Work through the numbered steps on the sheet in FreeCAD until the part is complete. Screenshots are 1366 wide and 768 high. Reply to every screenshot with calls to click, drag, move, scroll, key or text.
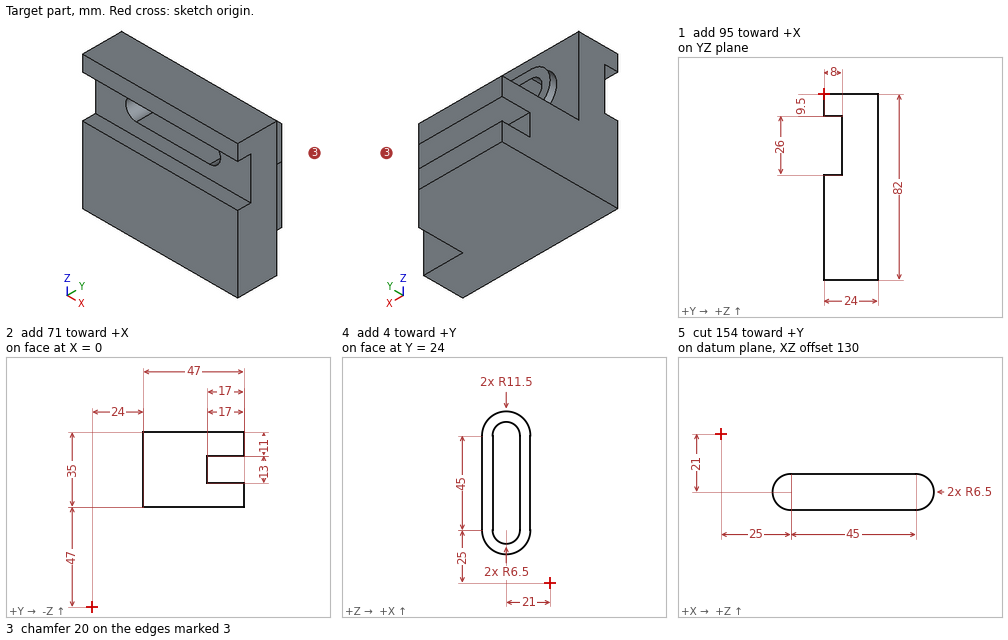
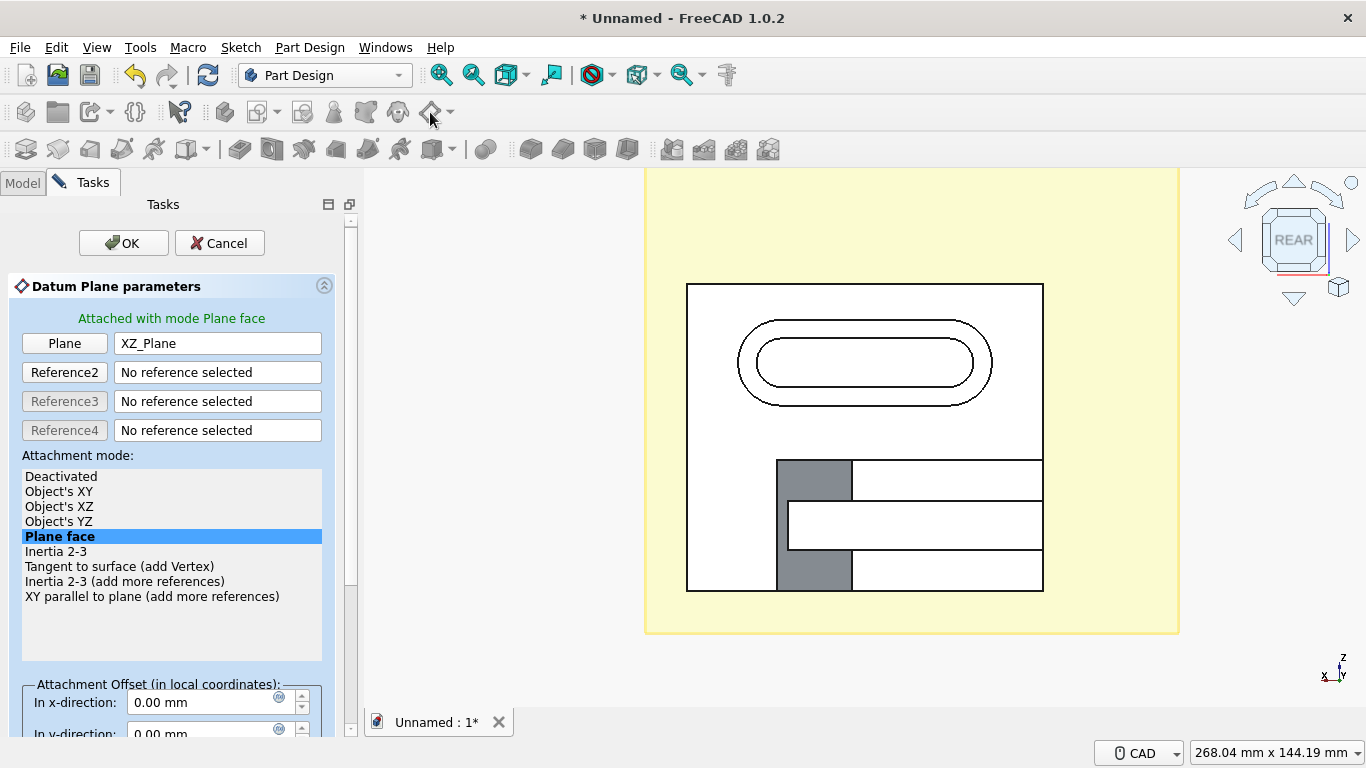
scroll(351, 475, down, 2)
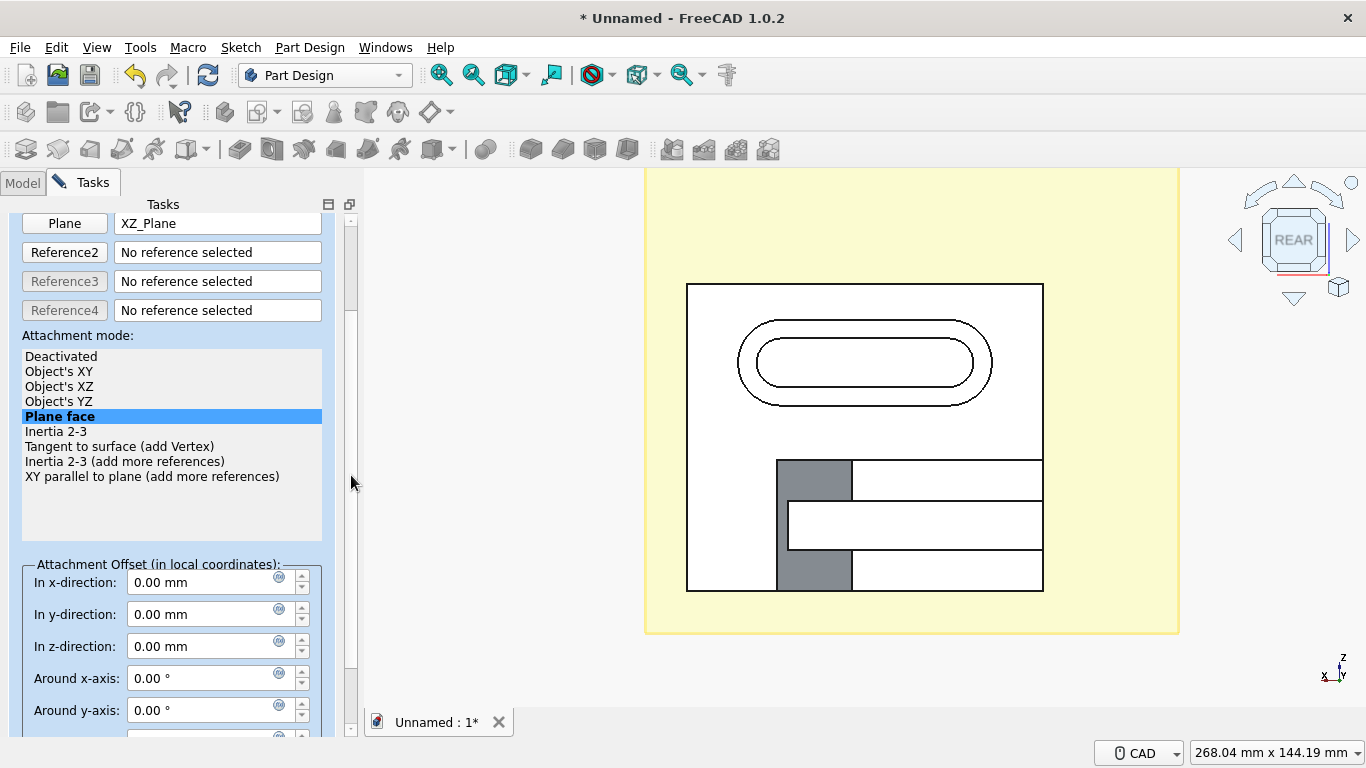
triple_click(210, 646)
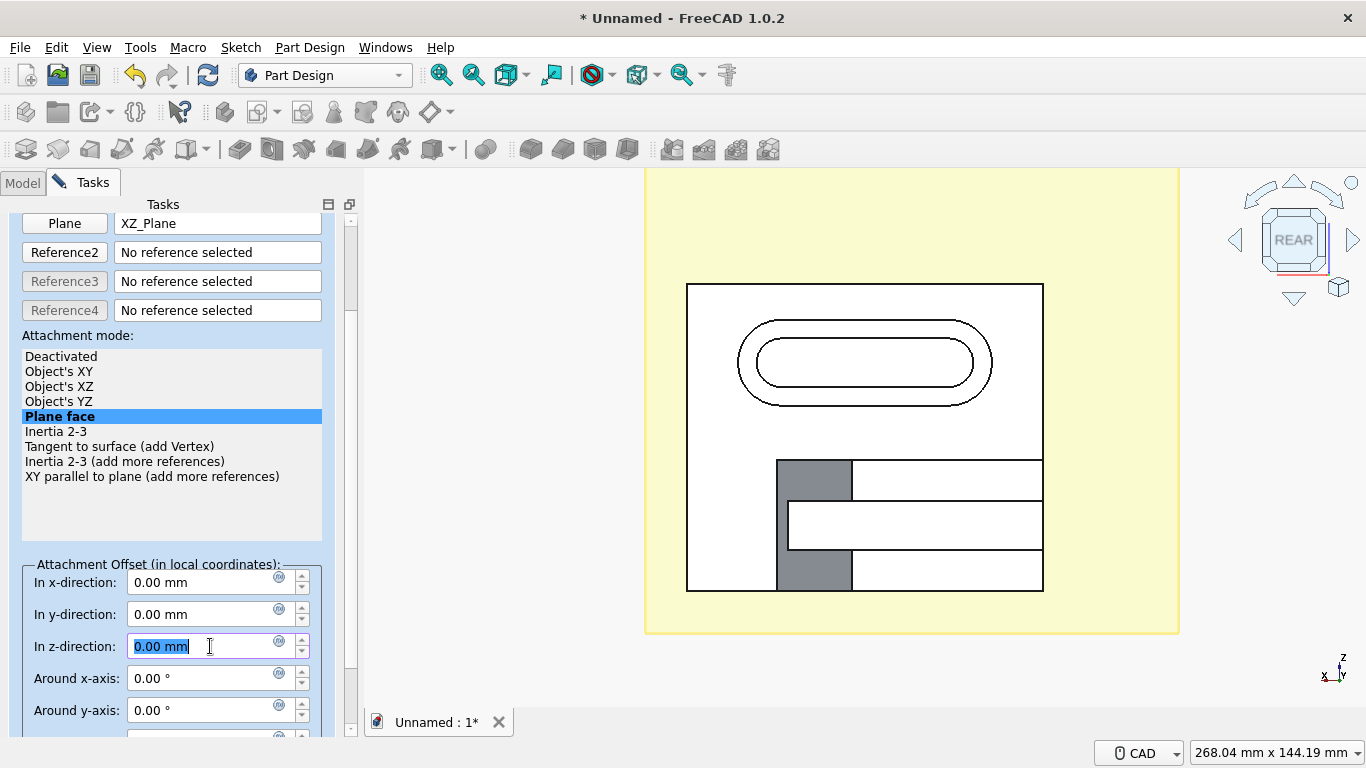
text(130)
key(Tab)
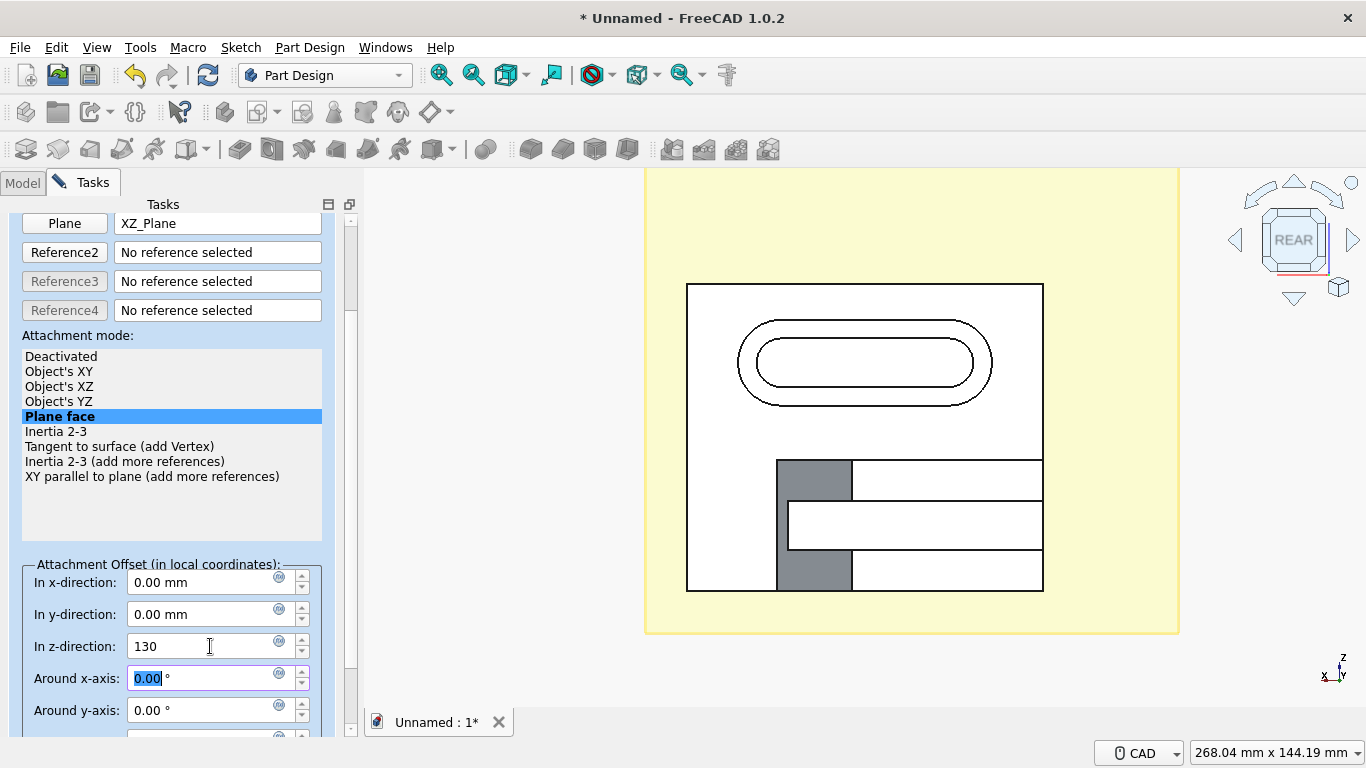
scroll(351, 475, up, 3)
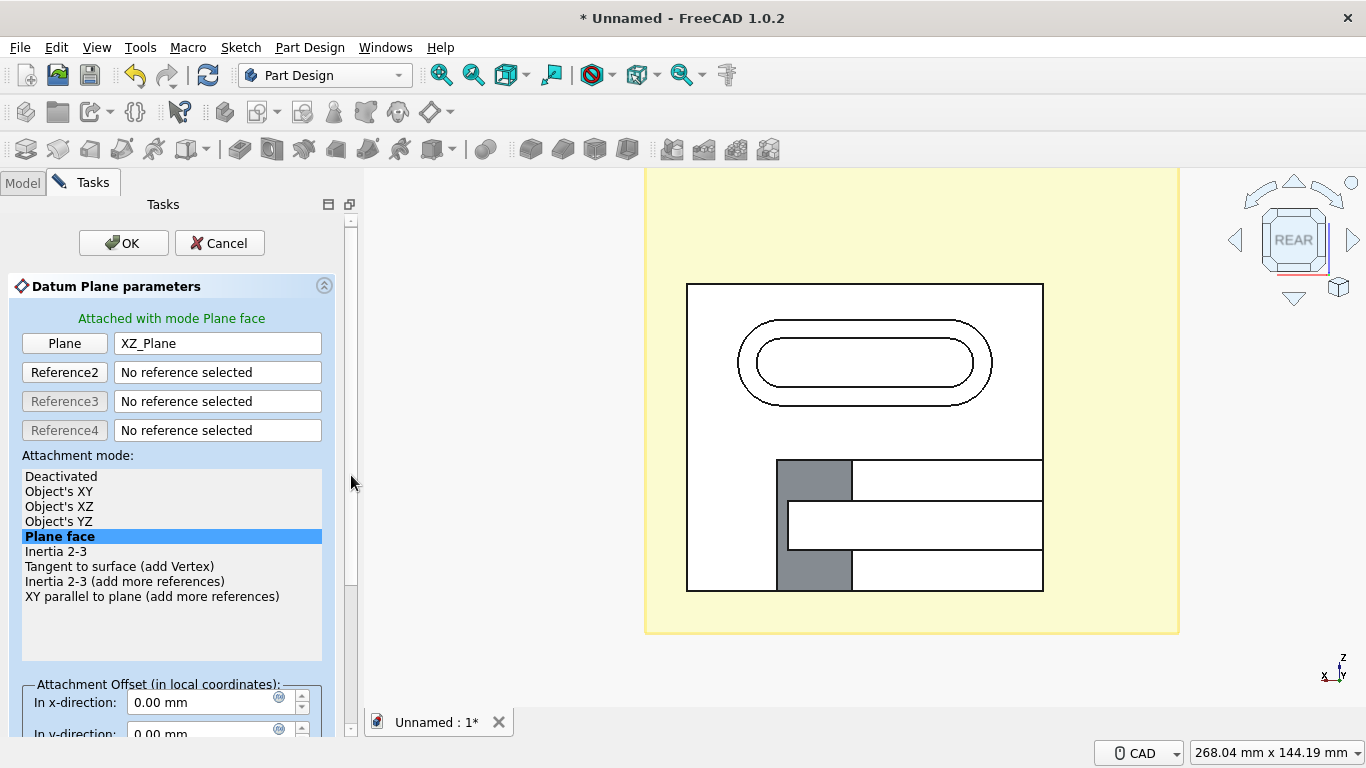
click(124, 243)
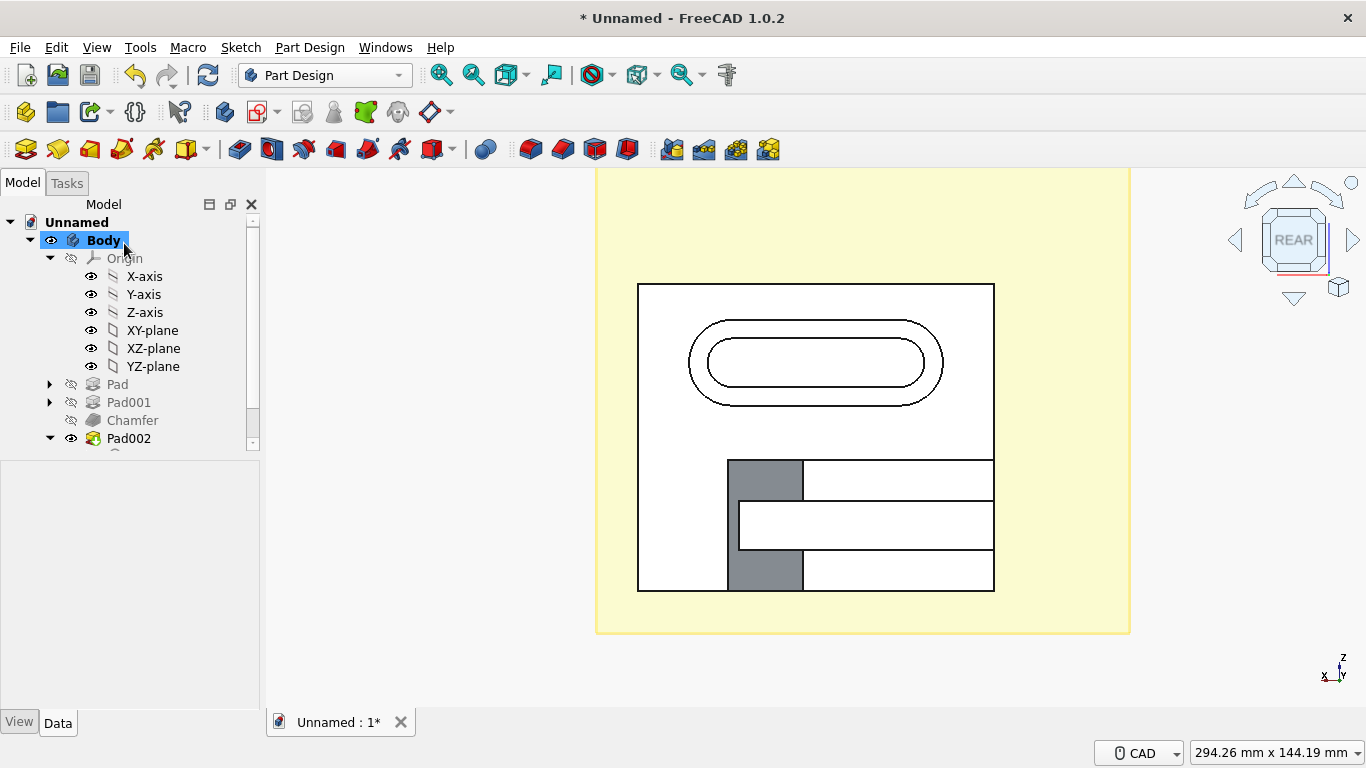
scroll(100, 326, down, 3)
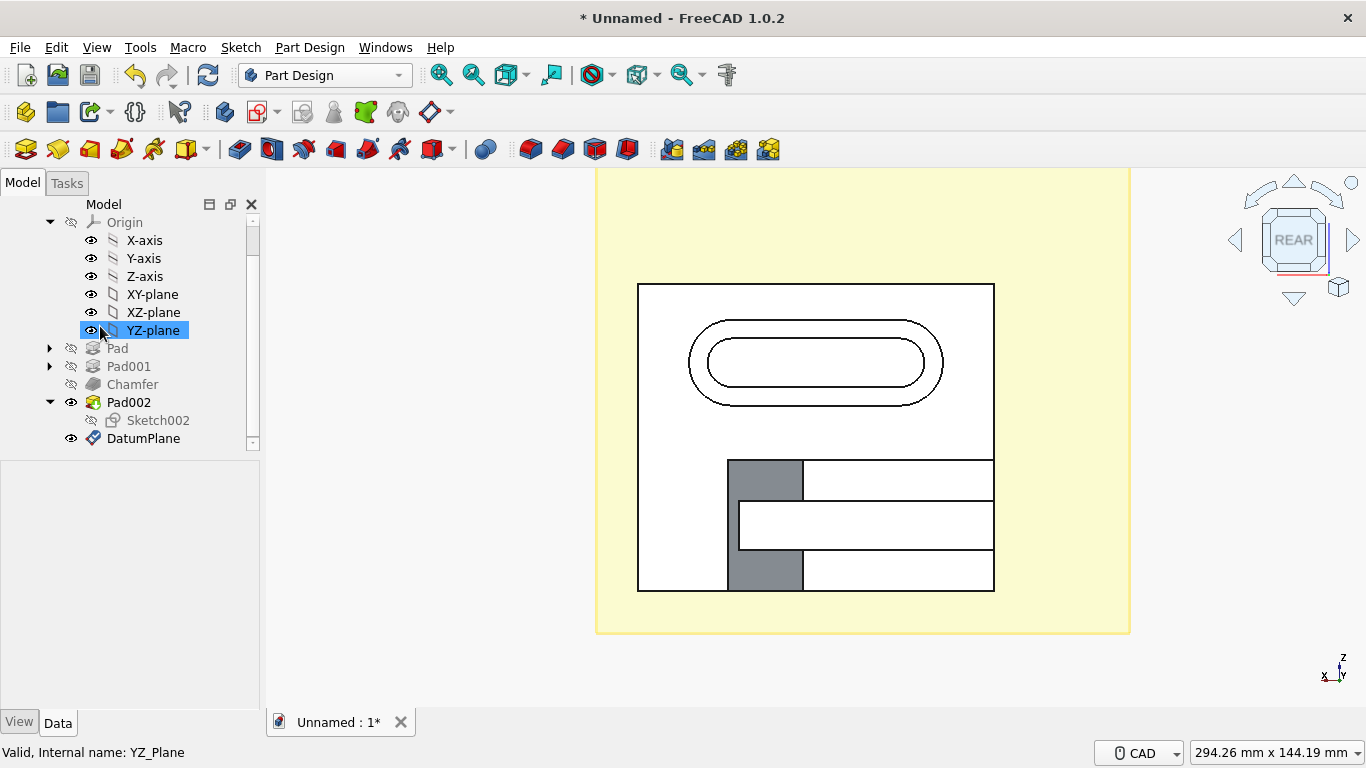
click(116, 438)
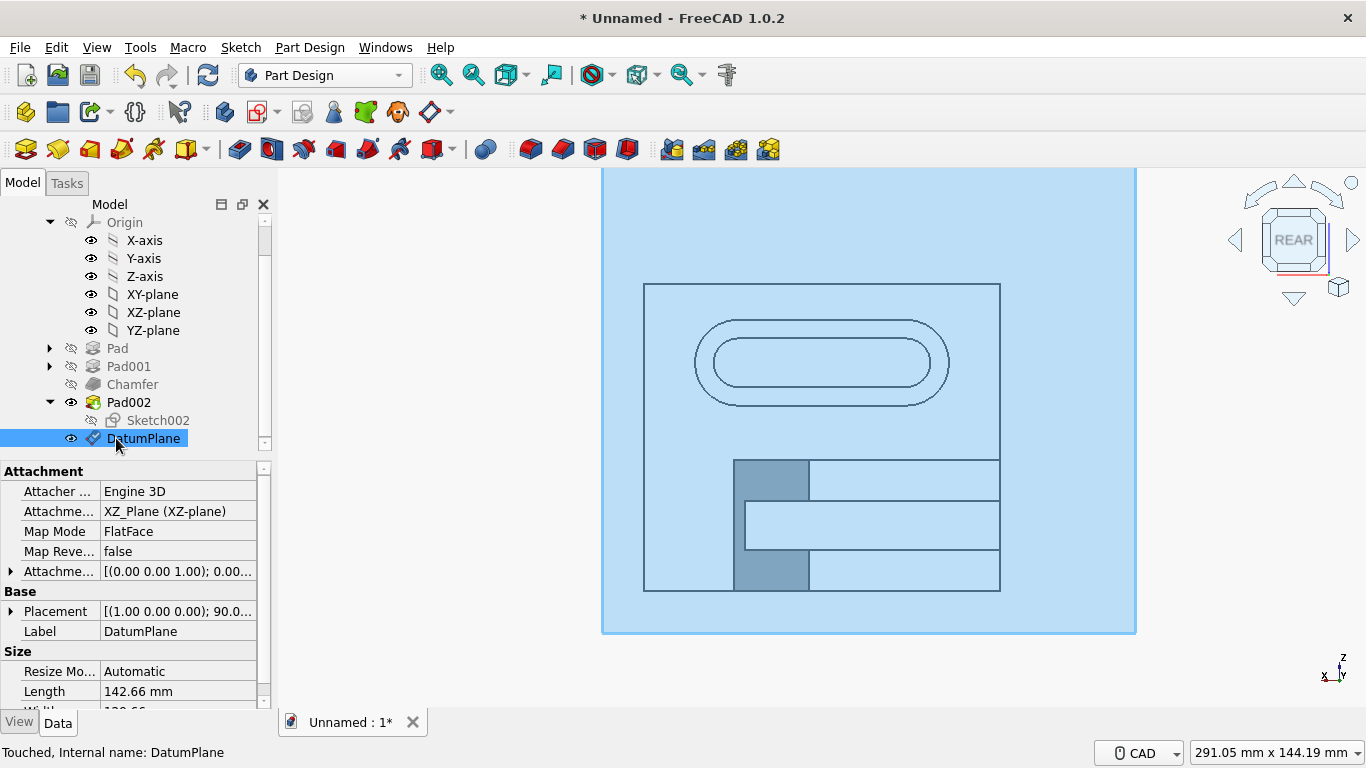
click(258, 112)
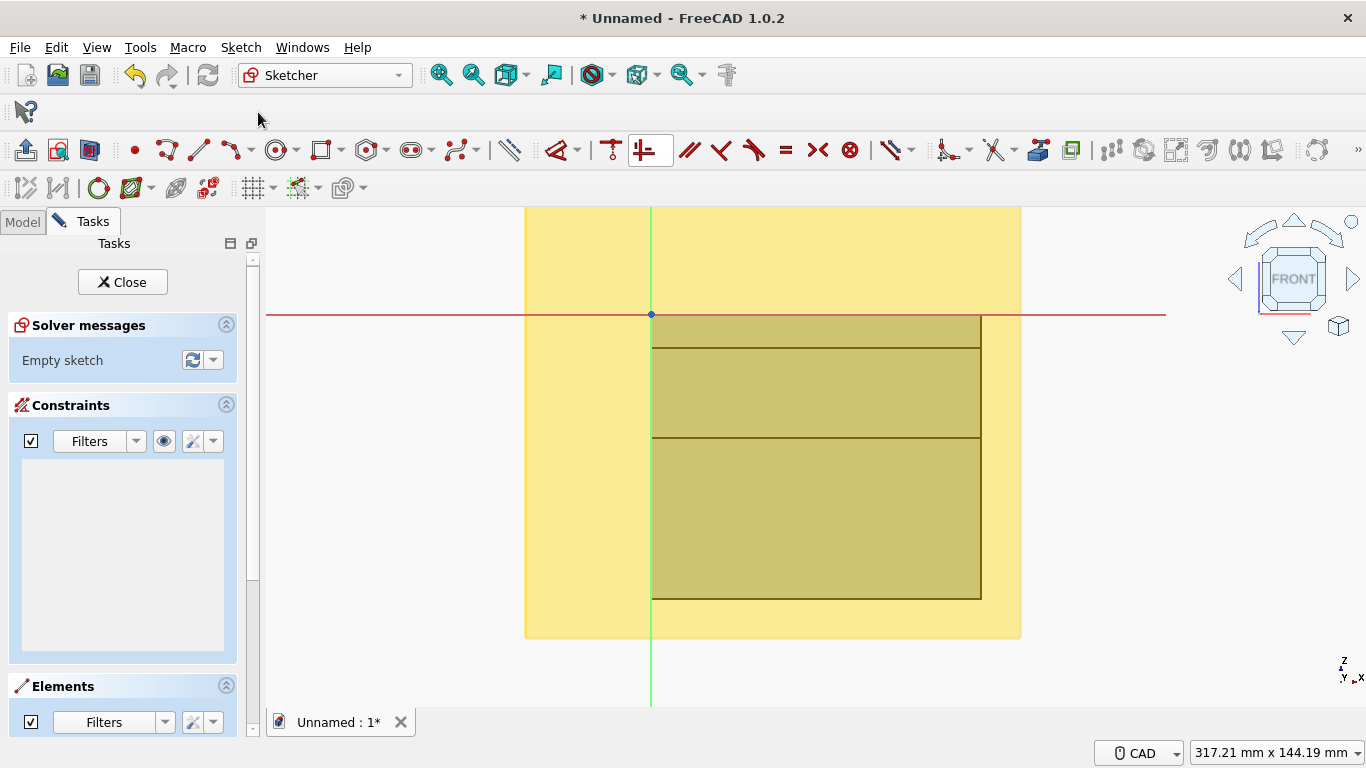
scroll(814, 285, up, 4)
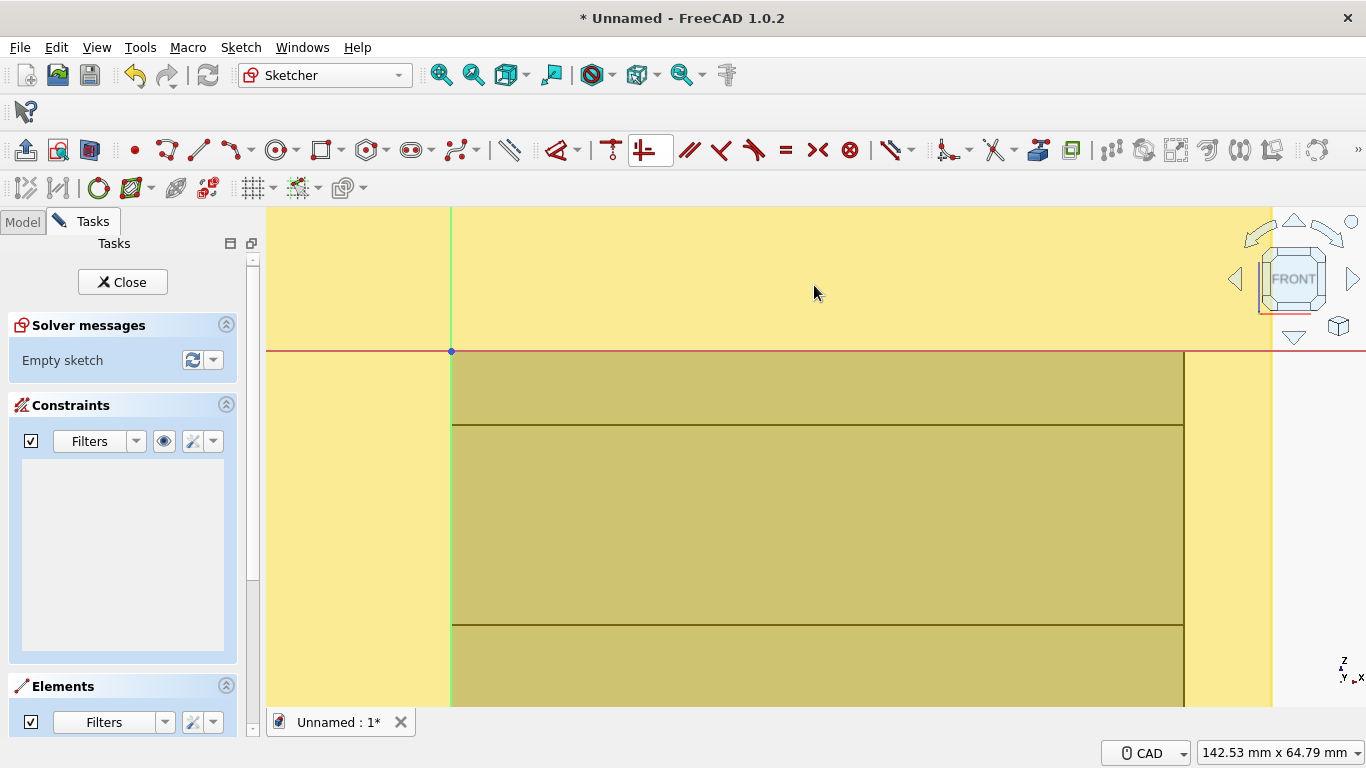
click(412, 150)